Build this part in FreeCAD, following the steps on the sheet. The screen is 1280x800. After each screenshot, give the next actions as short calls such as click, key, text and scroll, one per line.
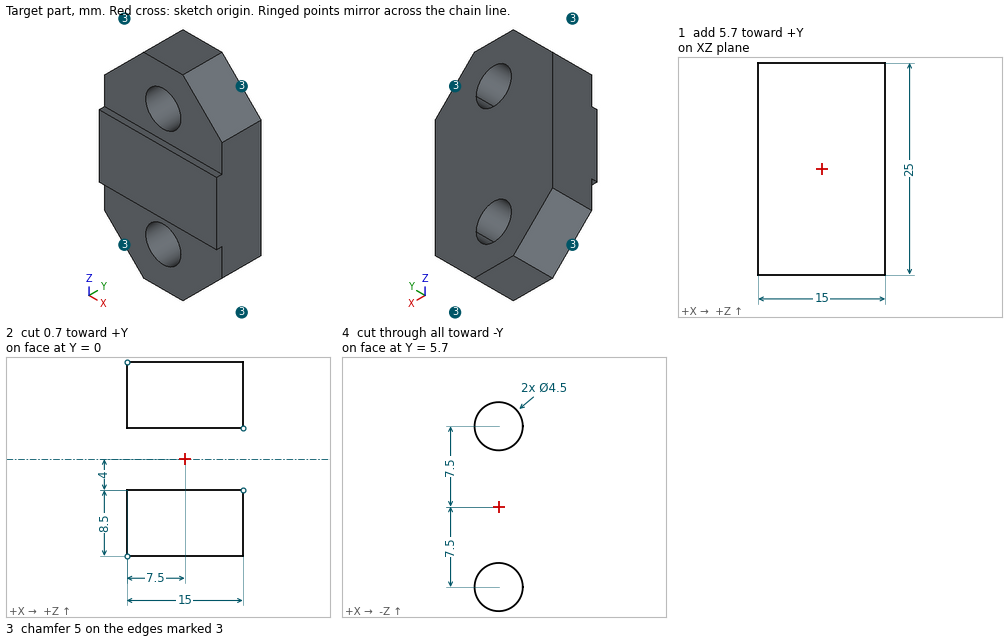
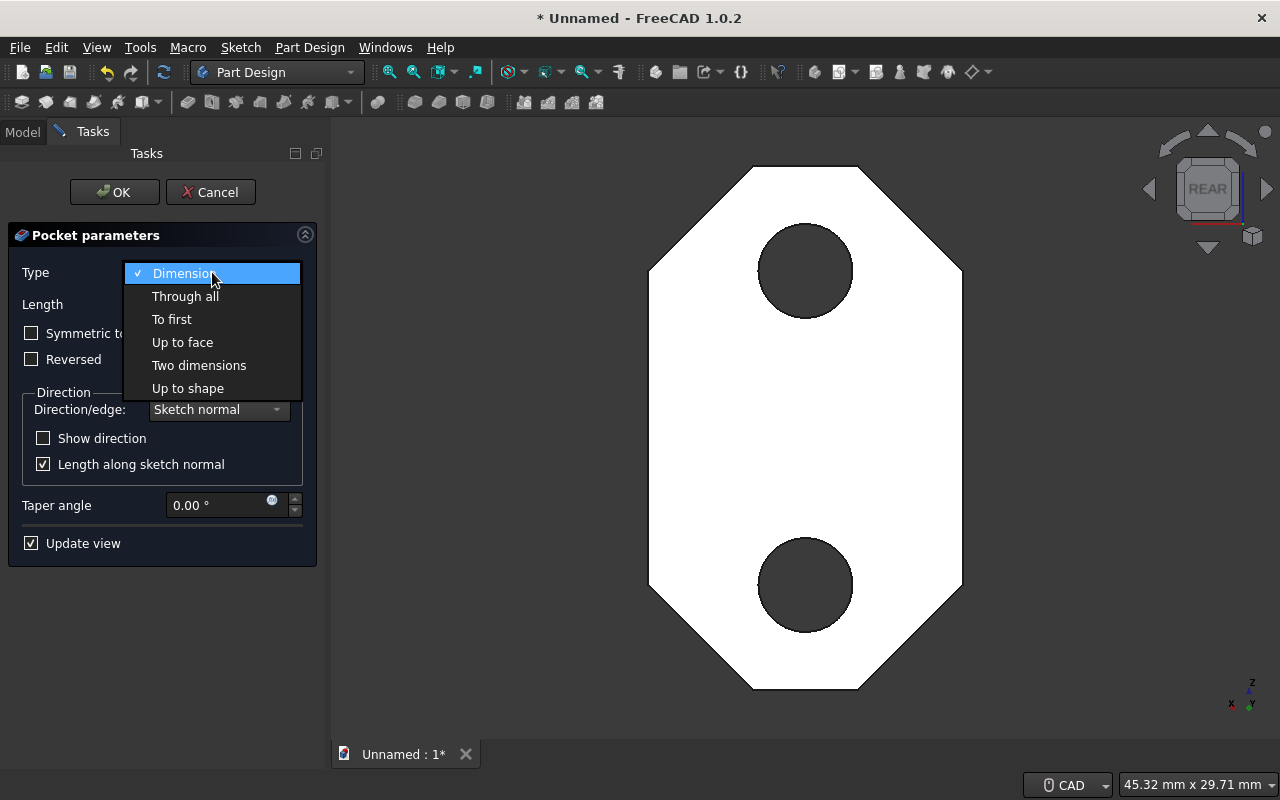
click(212, 296)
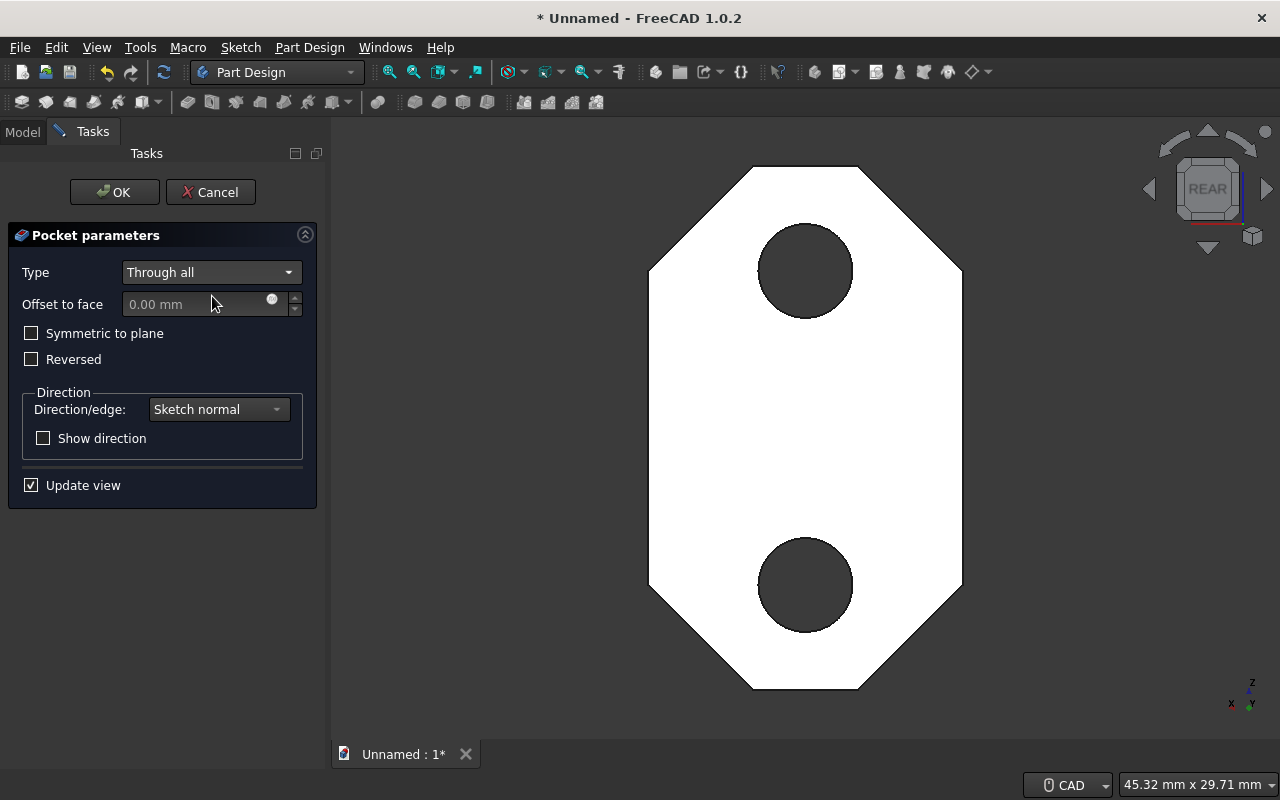
click(115, 192)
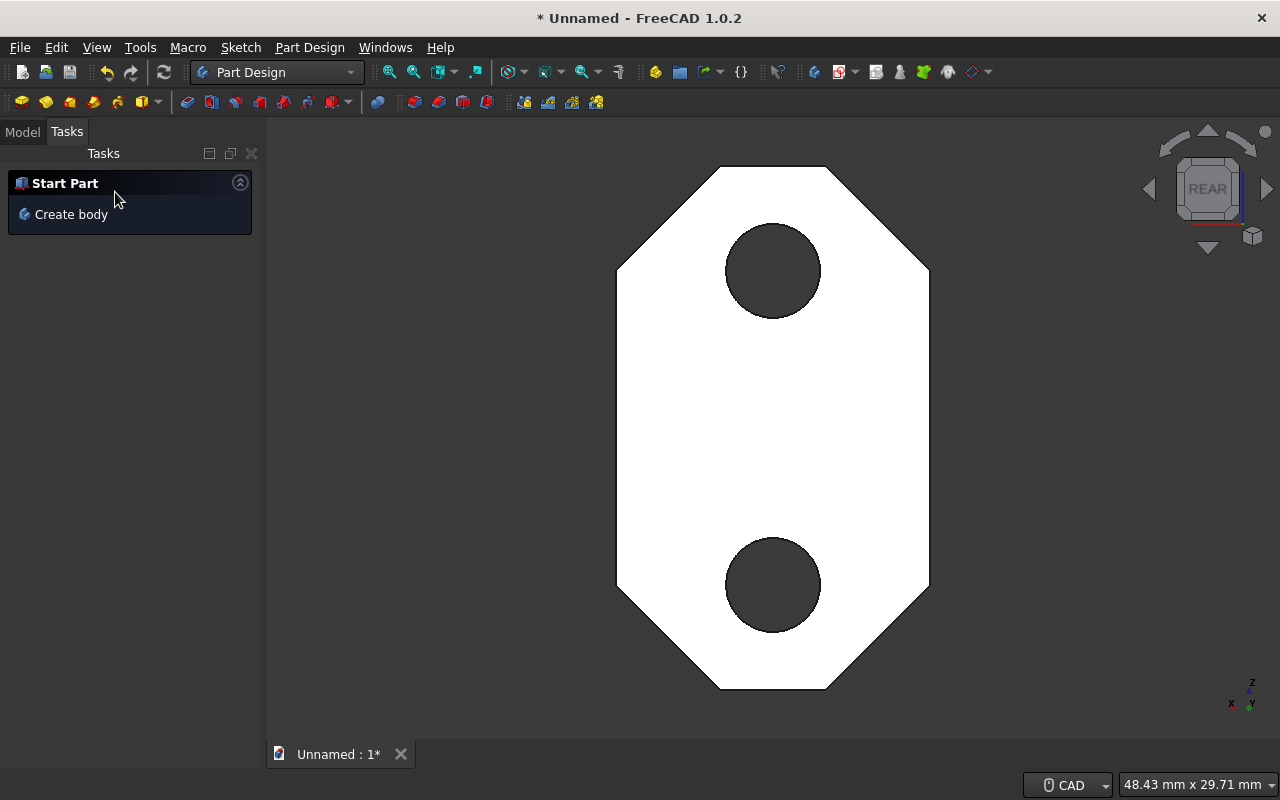
key(0)